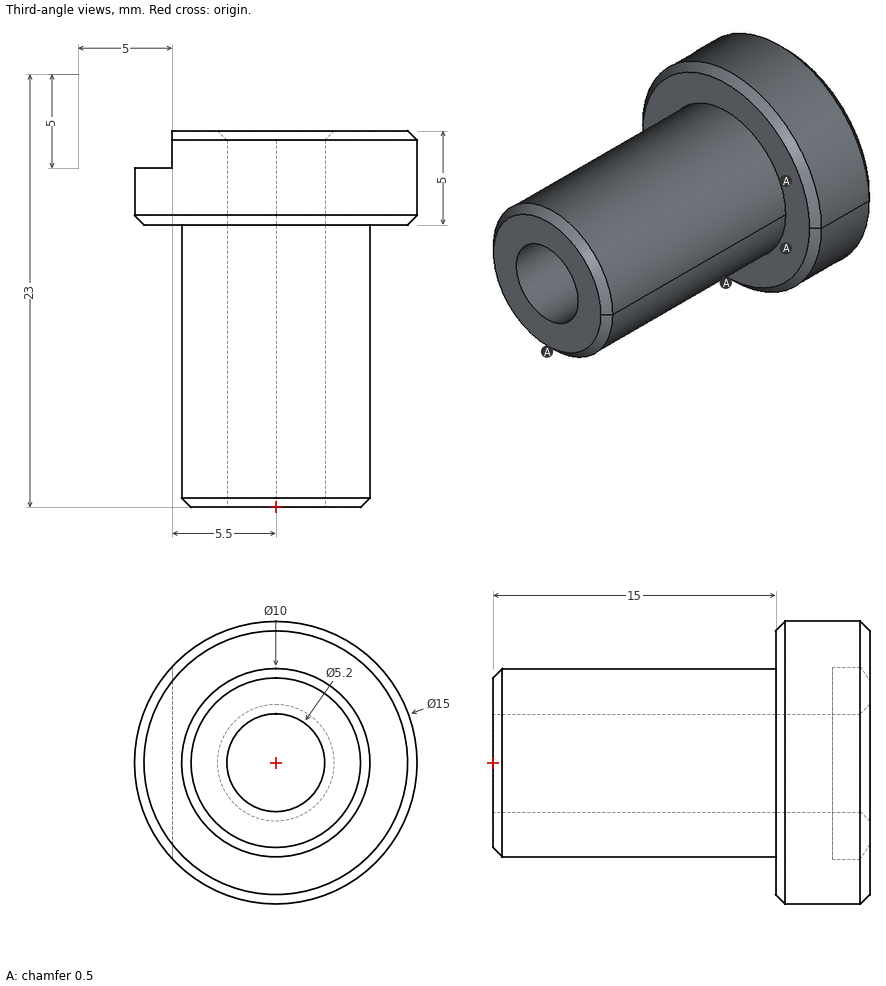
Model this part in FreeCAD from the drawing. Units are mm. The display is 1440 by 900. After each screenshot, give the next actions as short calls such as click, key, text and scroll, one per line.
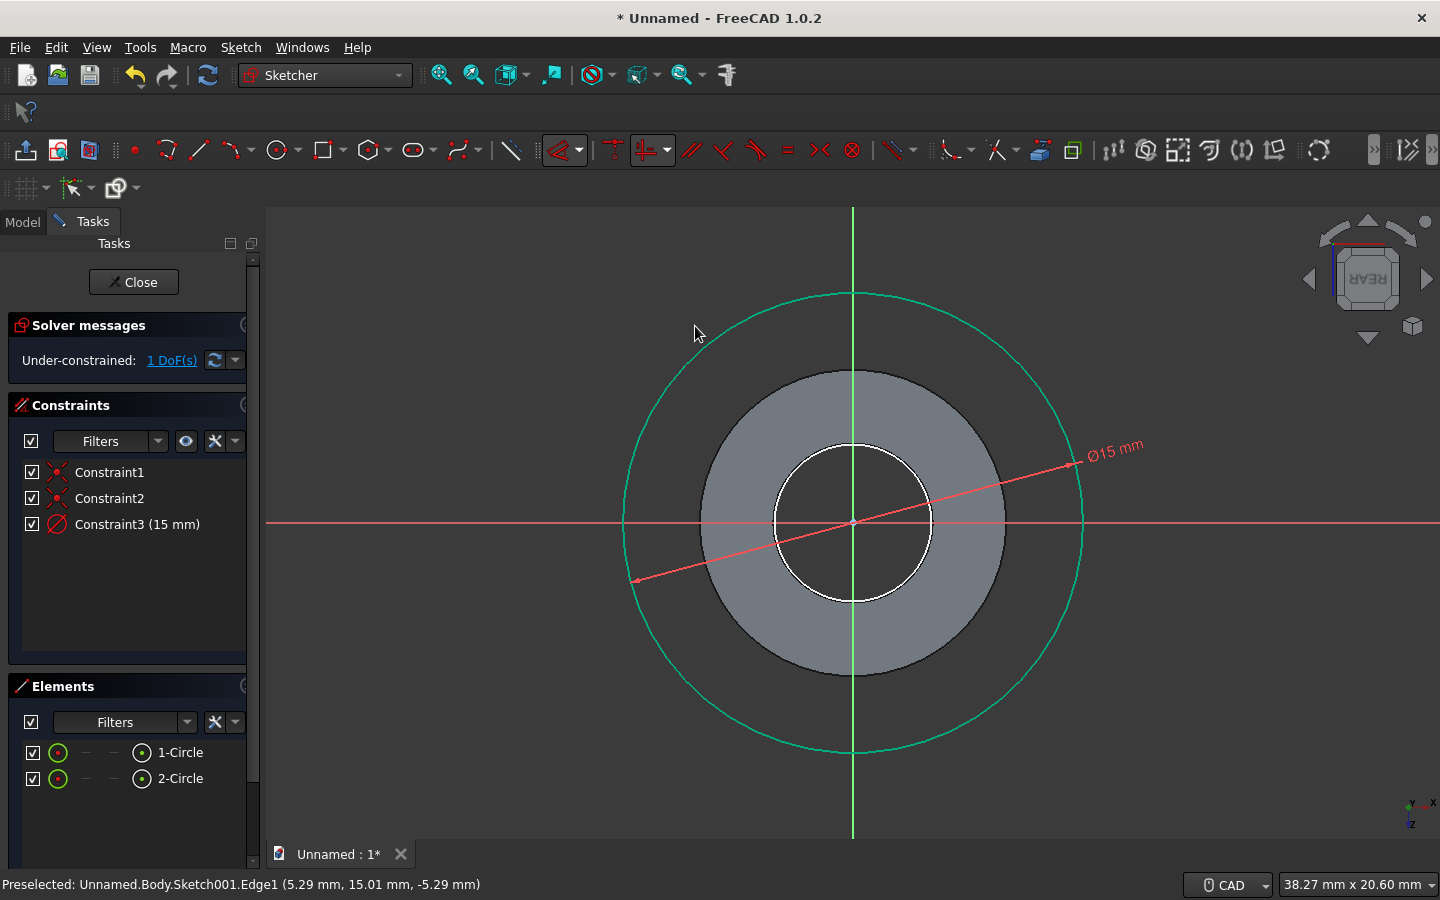
click(908, 467)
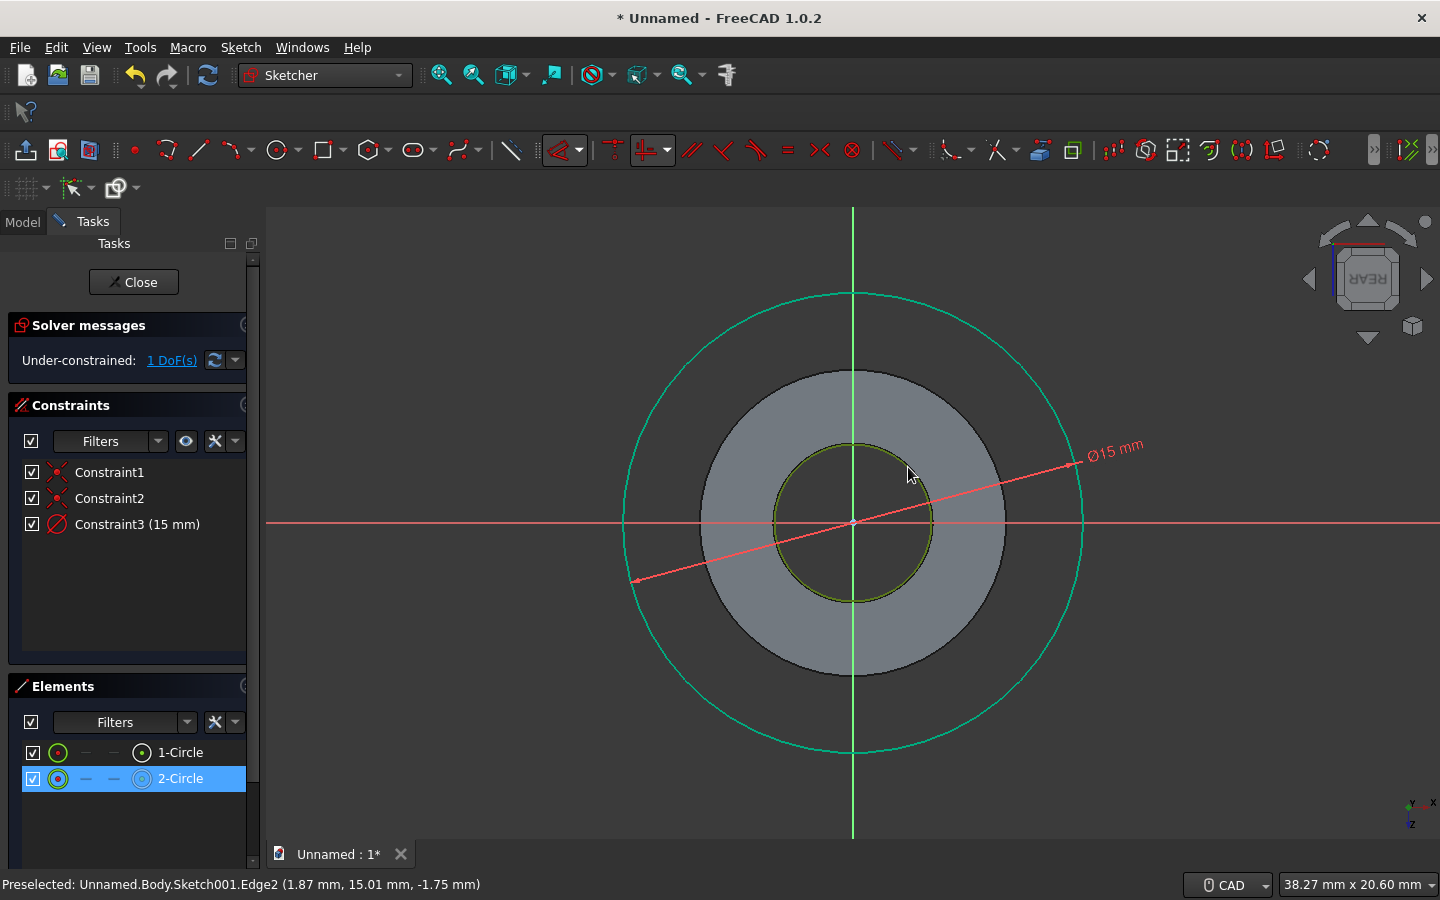
key(k)
key(o)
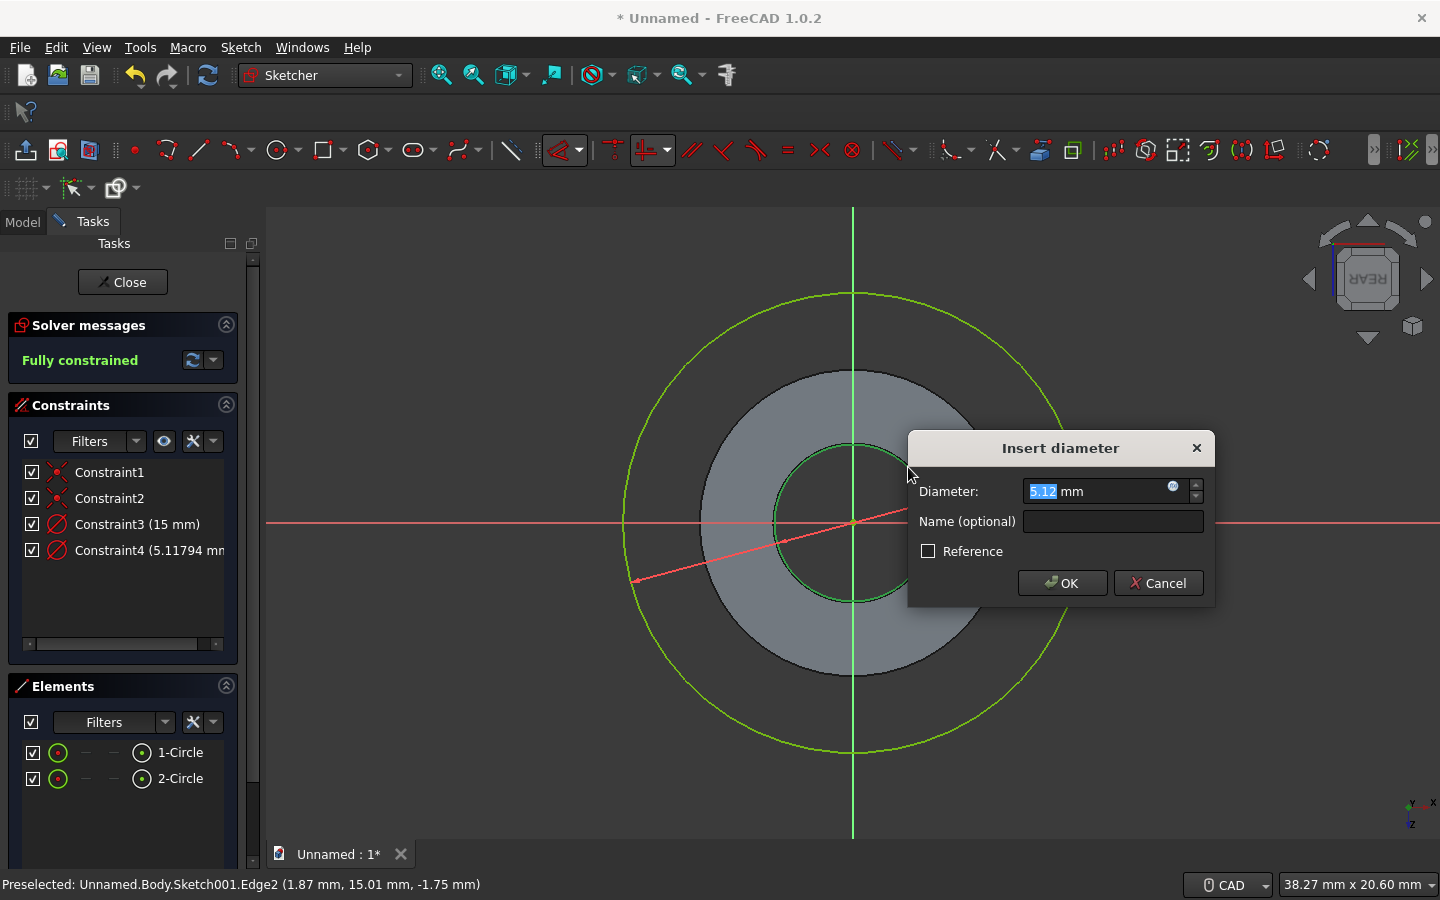
text(5.2)
key(Return)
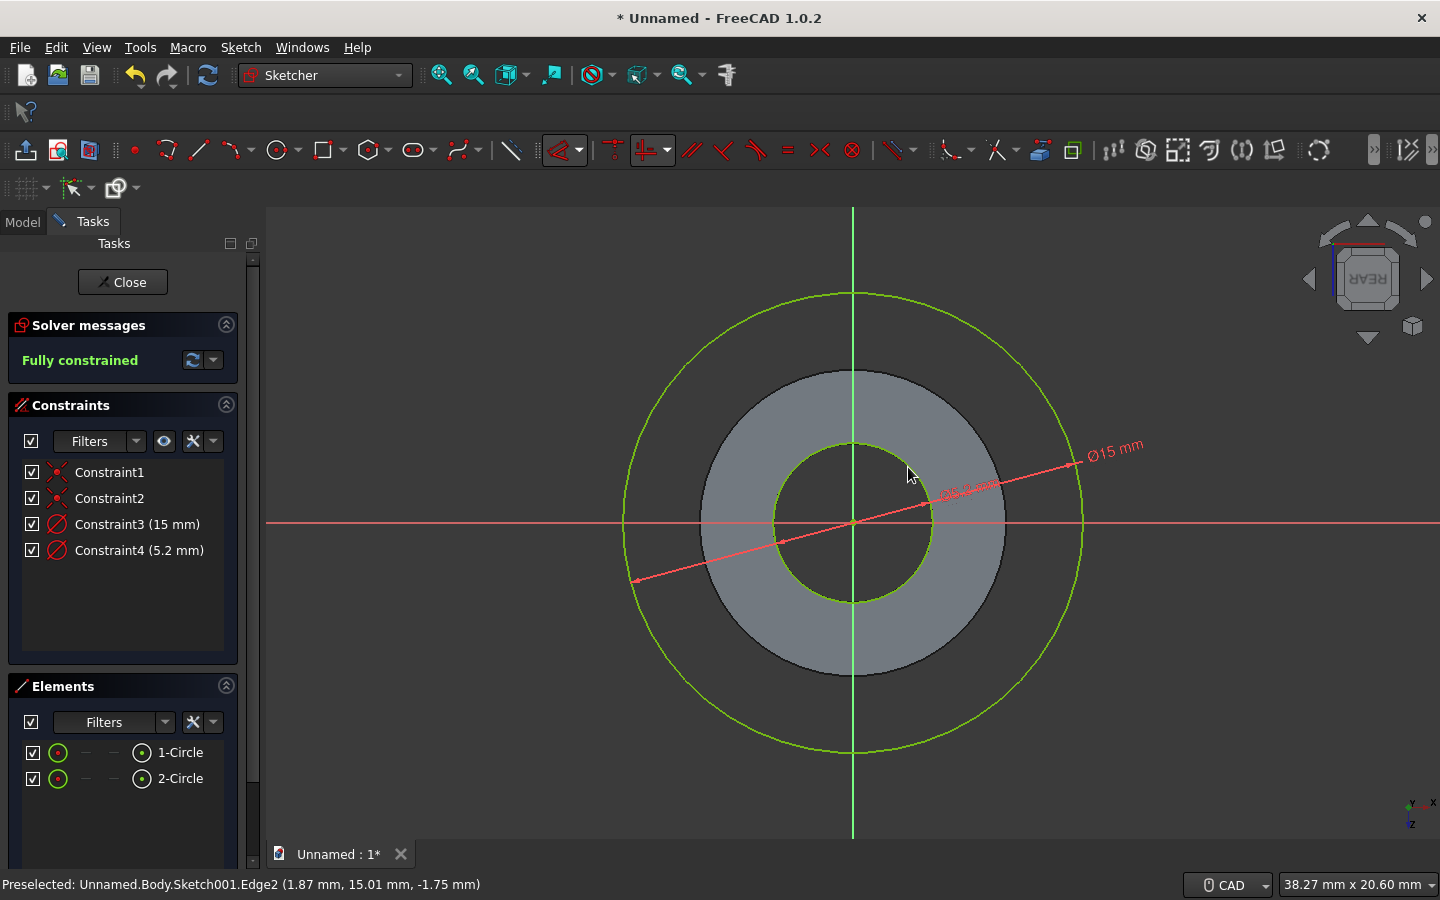
click(123, 282)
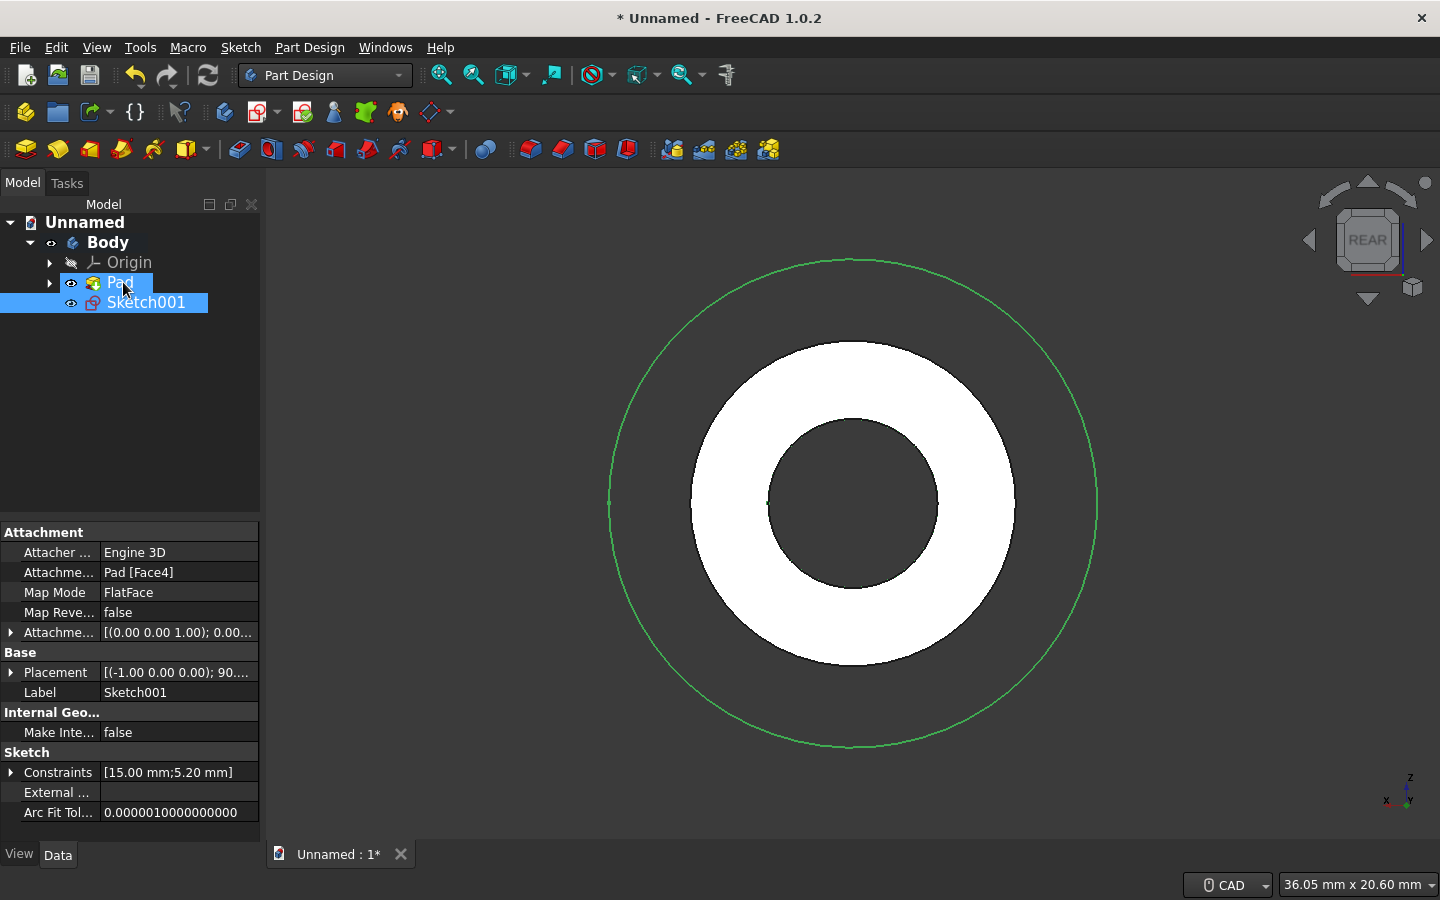
click(26, 150)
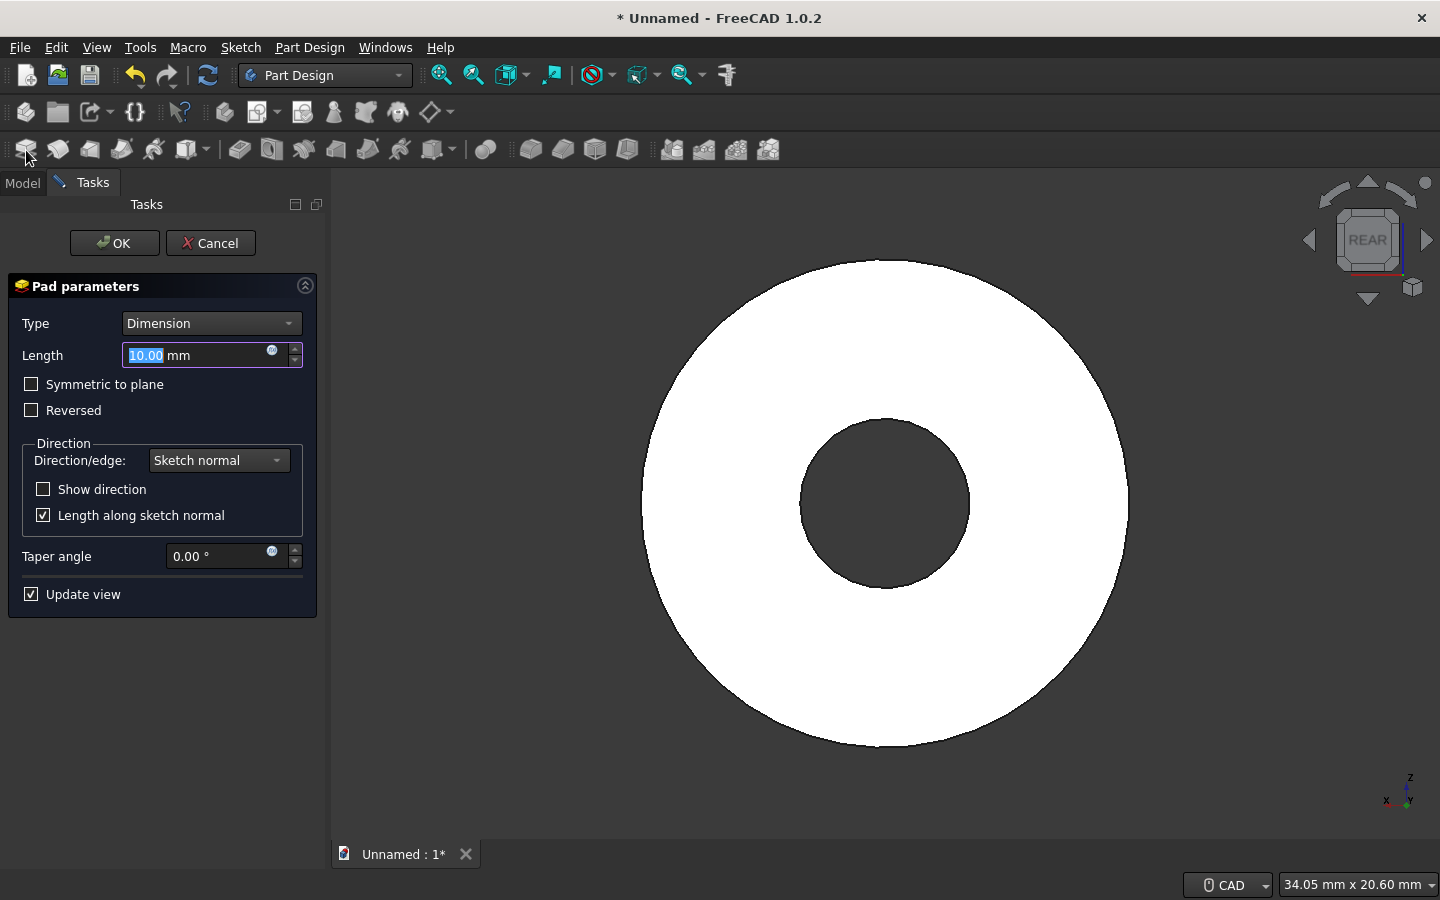
text(5)
key(Tab)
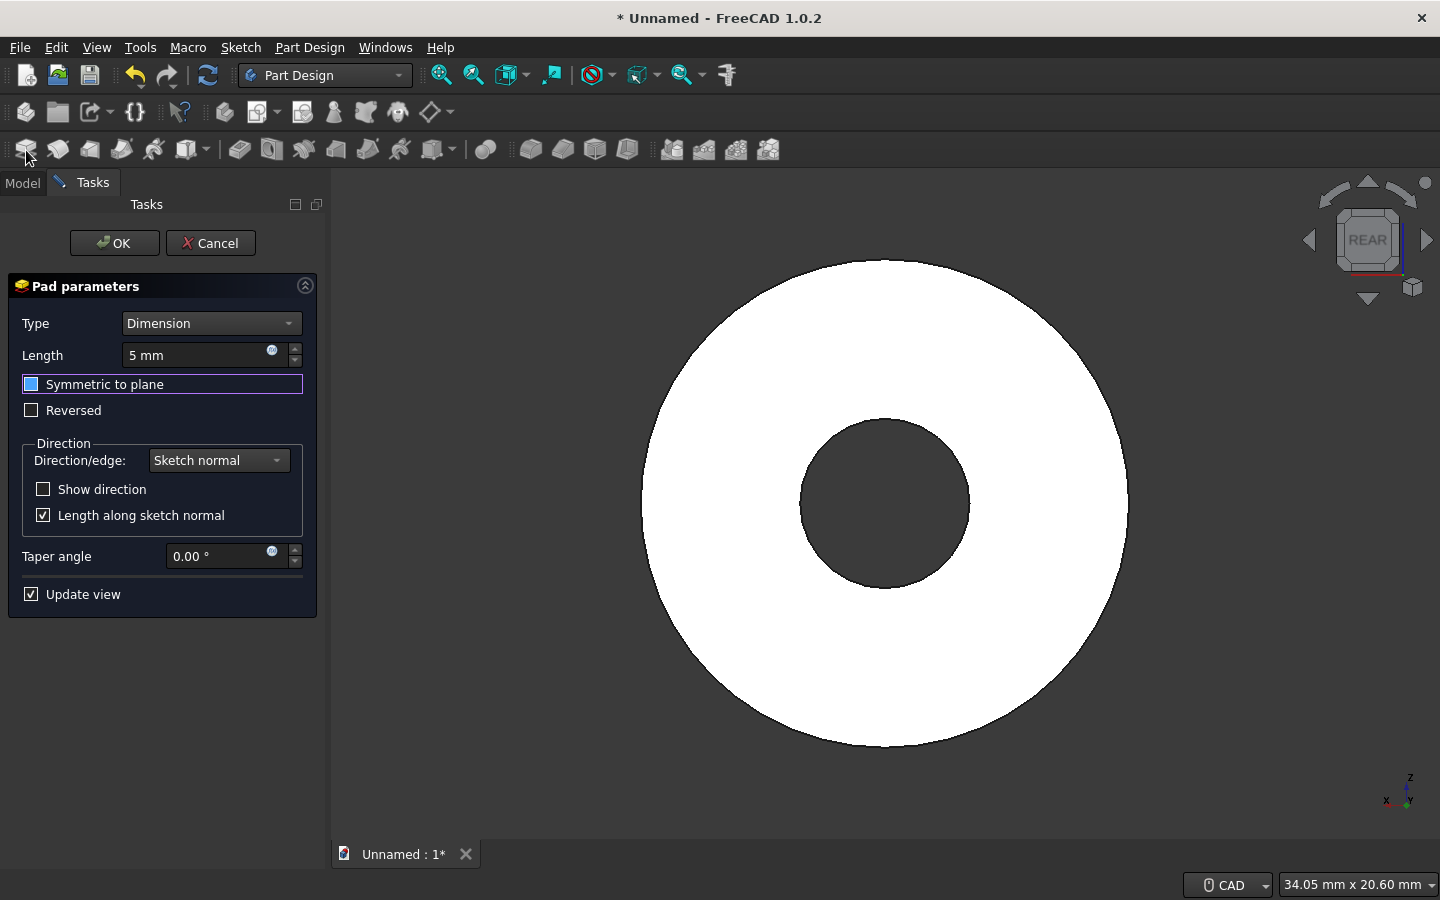
click(115, 243)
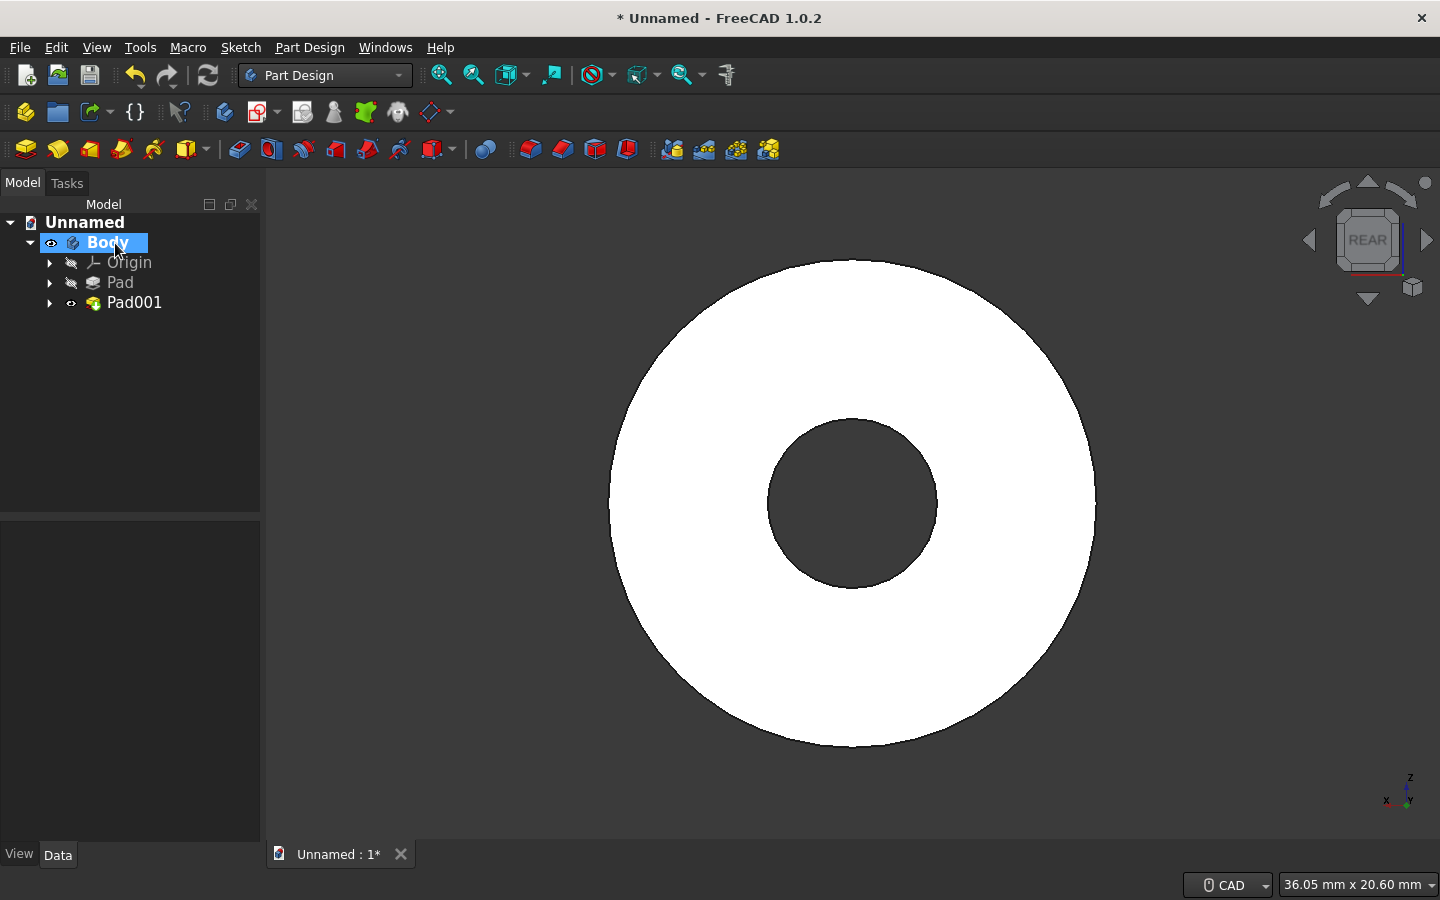
click(1097, 503)